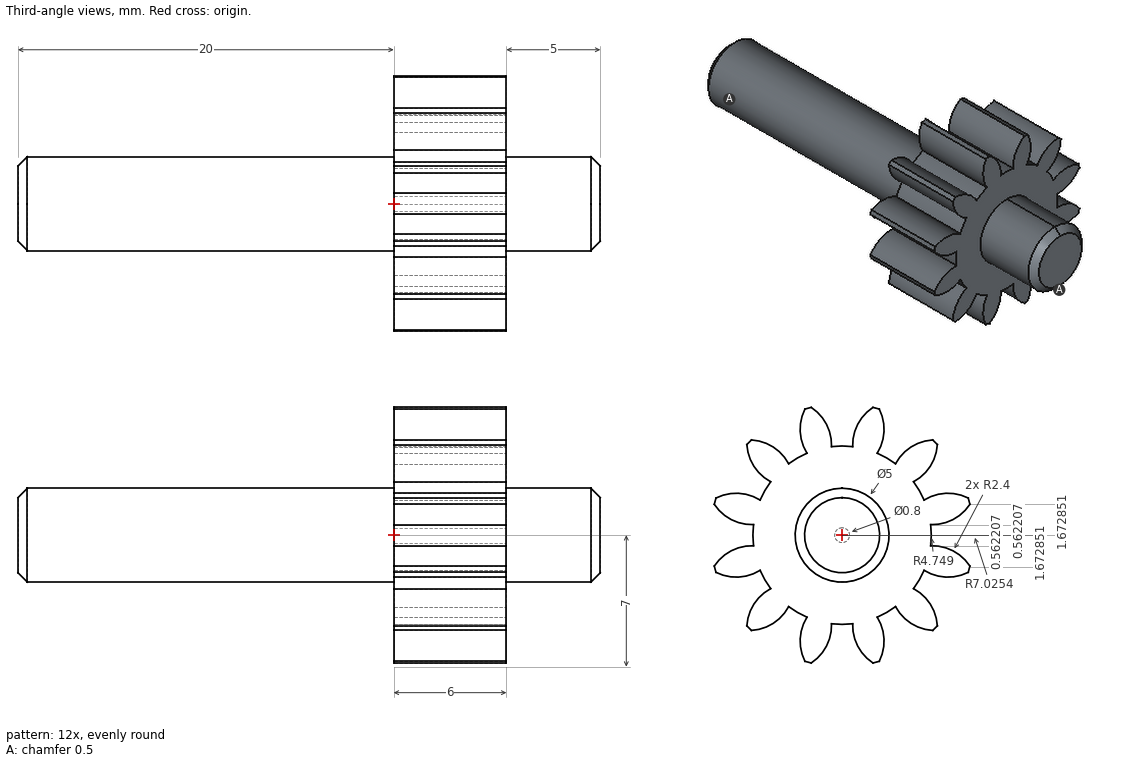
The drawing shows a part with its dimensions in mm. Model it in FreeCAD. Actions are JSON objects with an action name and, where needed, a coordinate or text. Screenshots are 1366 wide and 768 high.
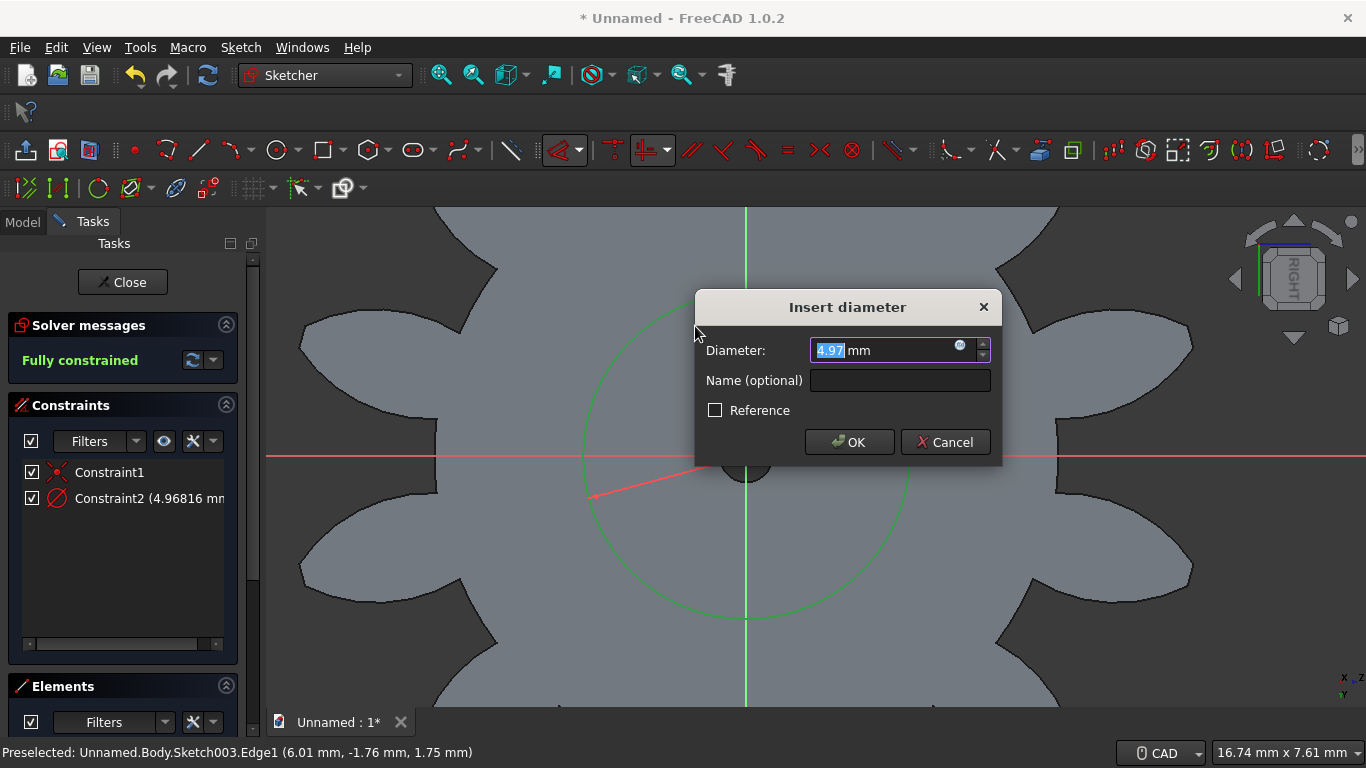
{"action": "type", "text": "5"}
{"action": "key", "text": "Return"}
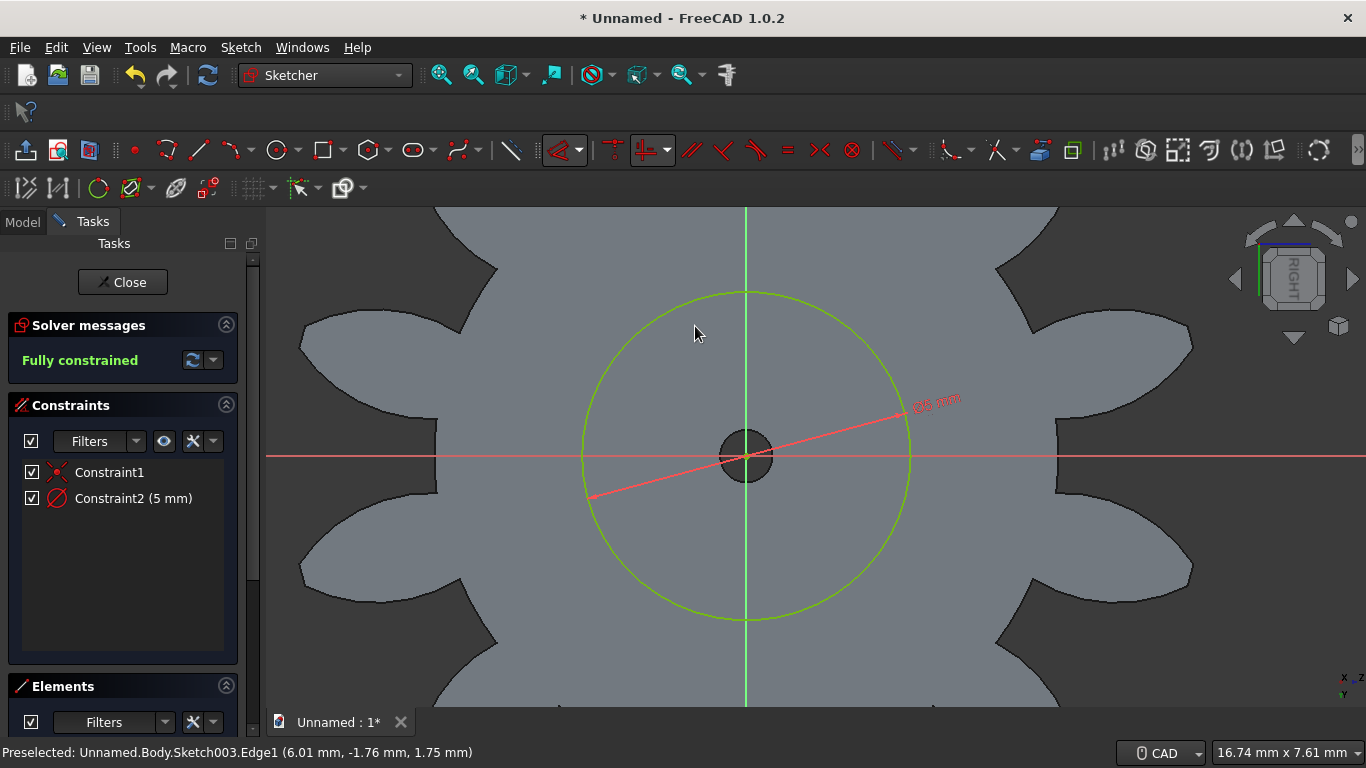
{"action": "left_click", "coordinate": [123, 282]}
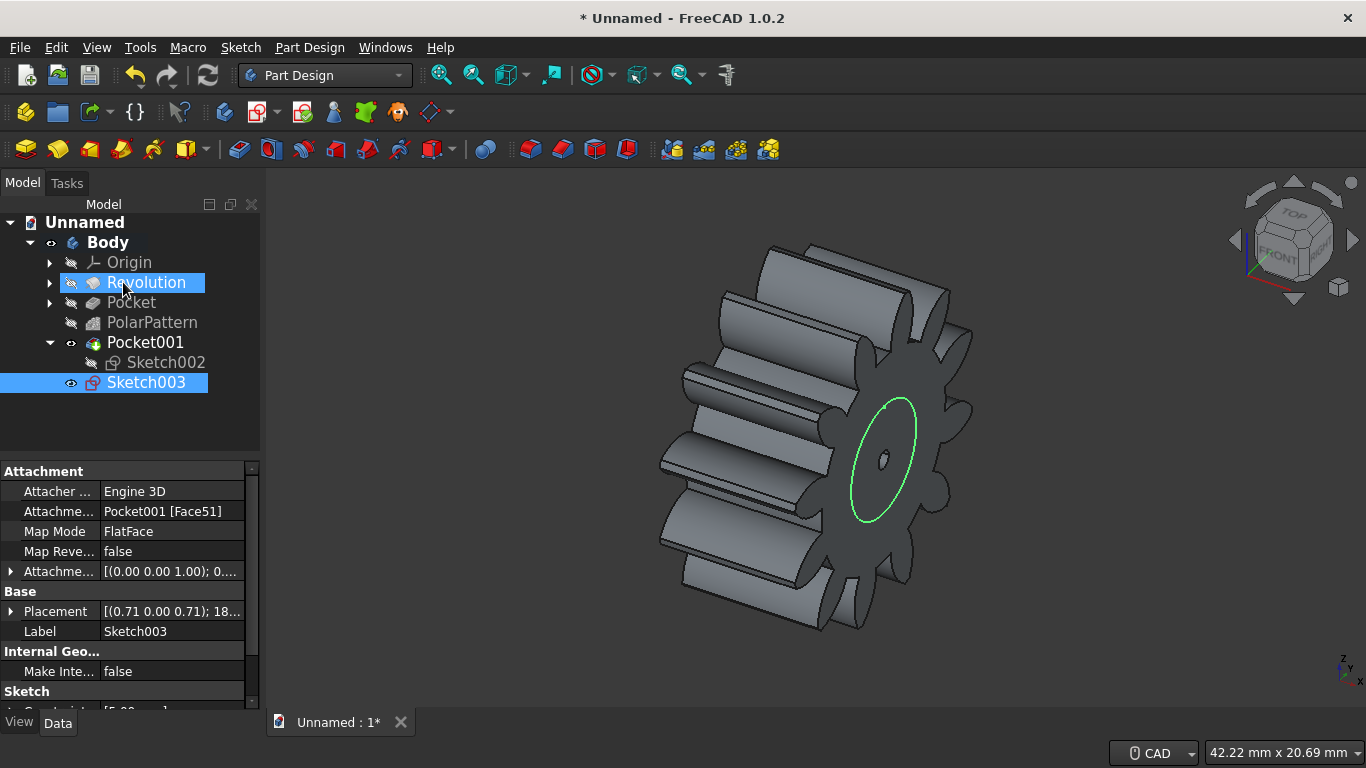
{"action": "left_click", "coordinate": [26, 150]}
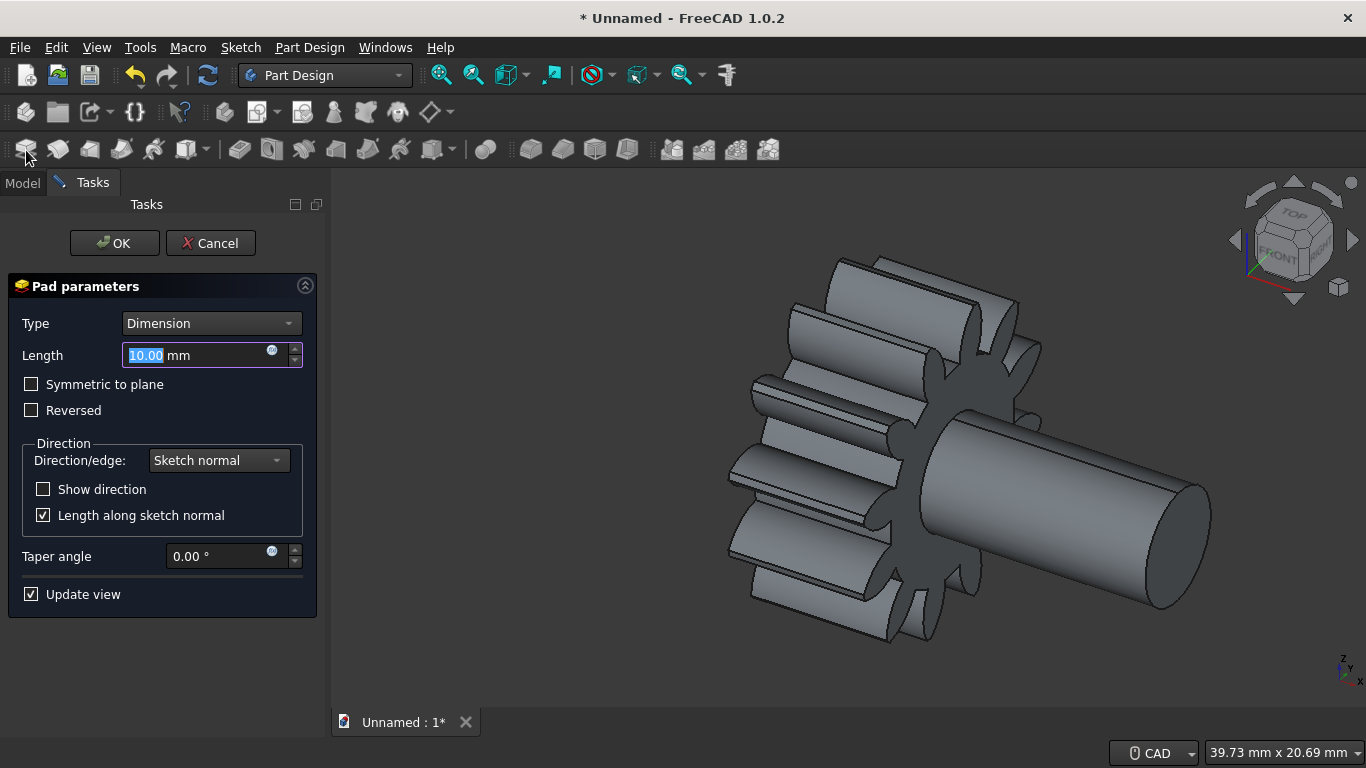
{"action": "type", "text": "5"}
{"action": "key", "text": "Tab"}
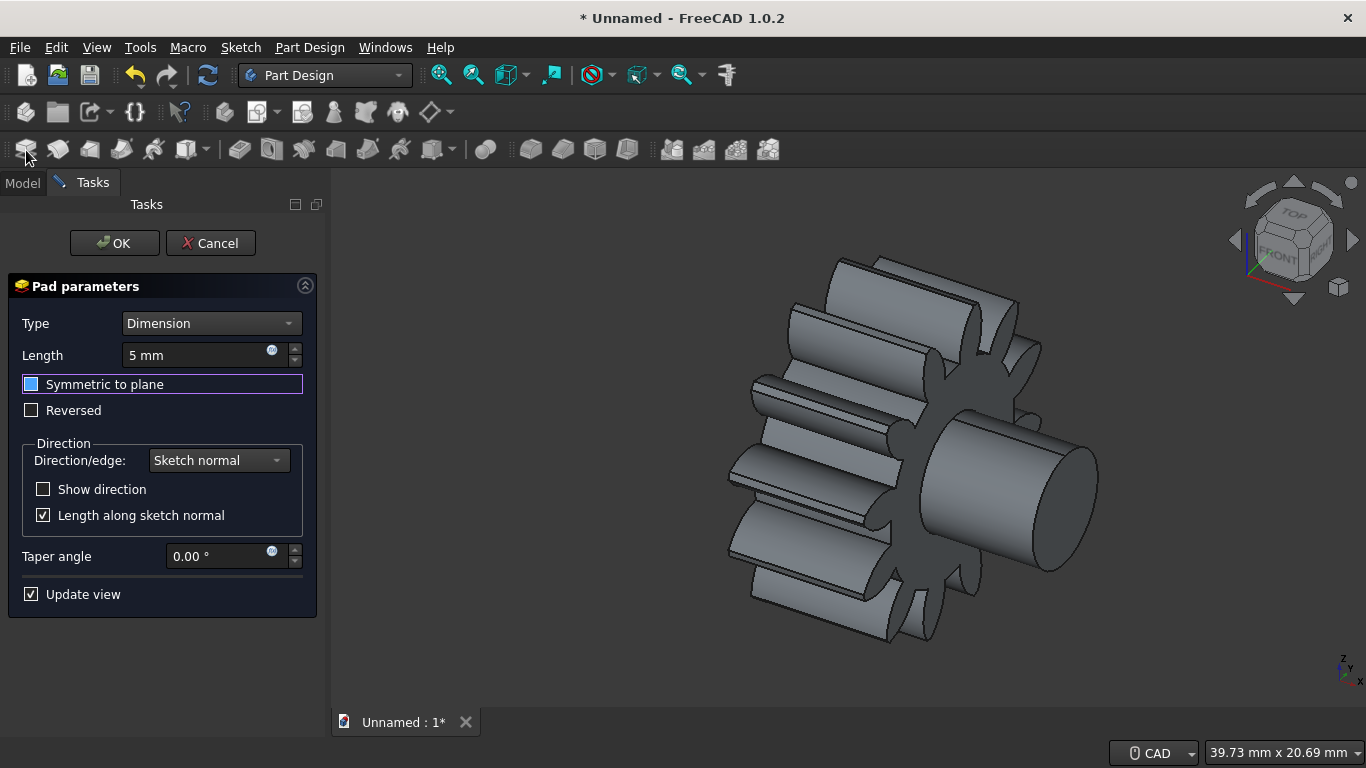
{"action": "left_click", "coordinate": [115, 243]}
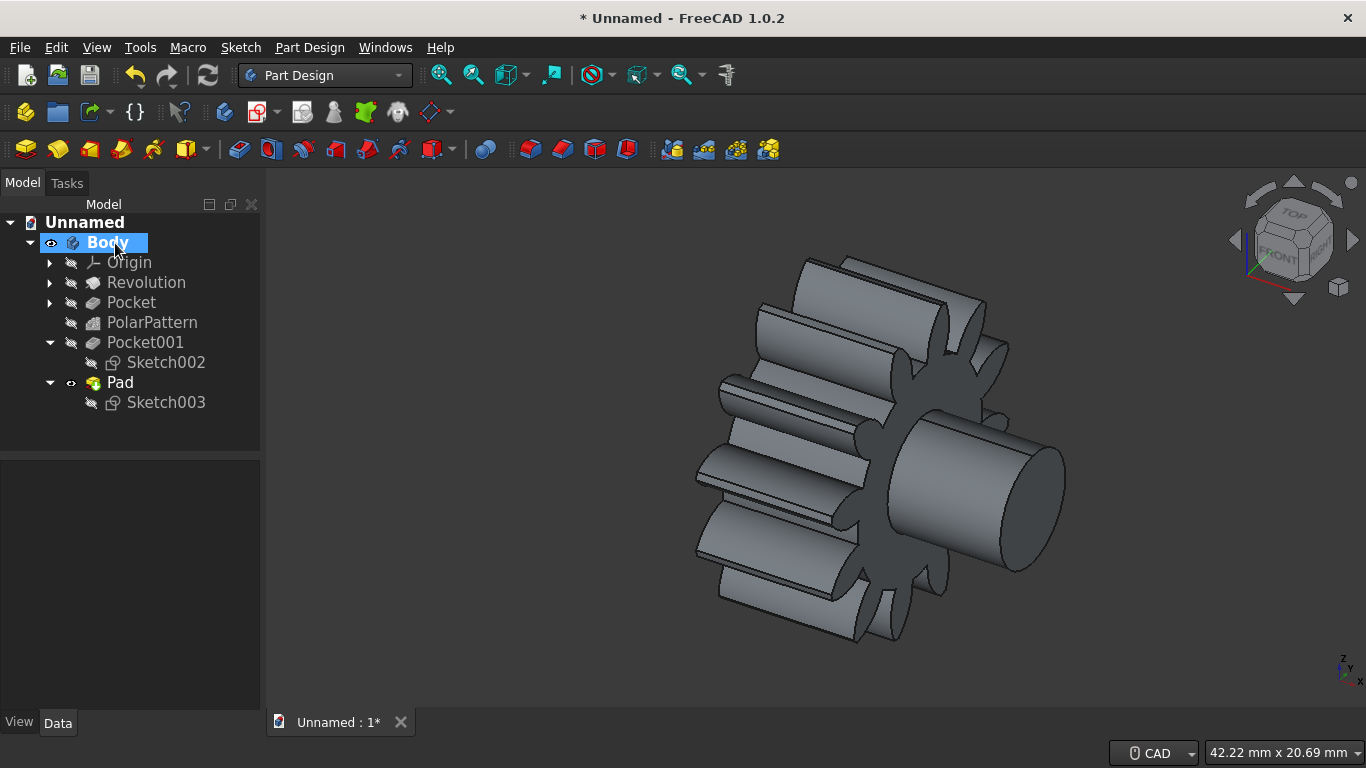
{"action": "left_click", "coordinate": [442, 76]}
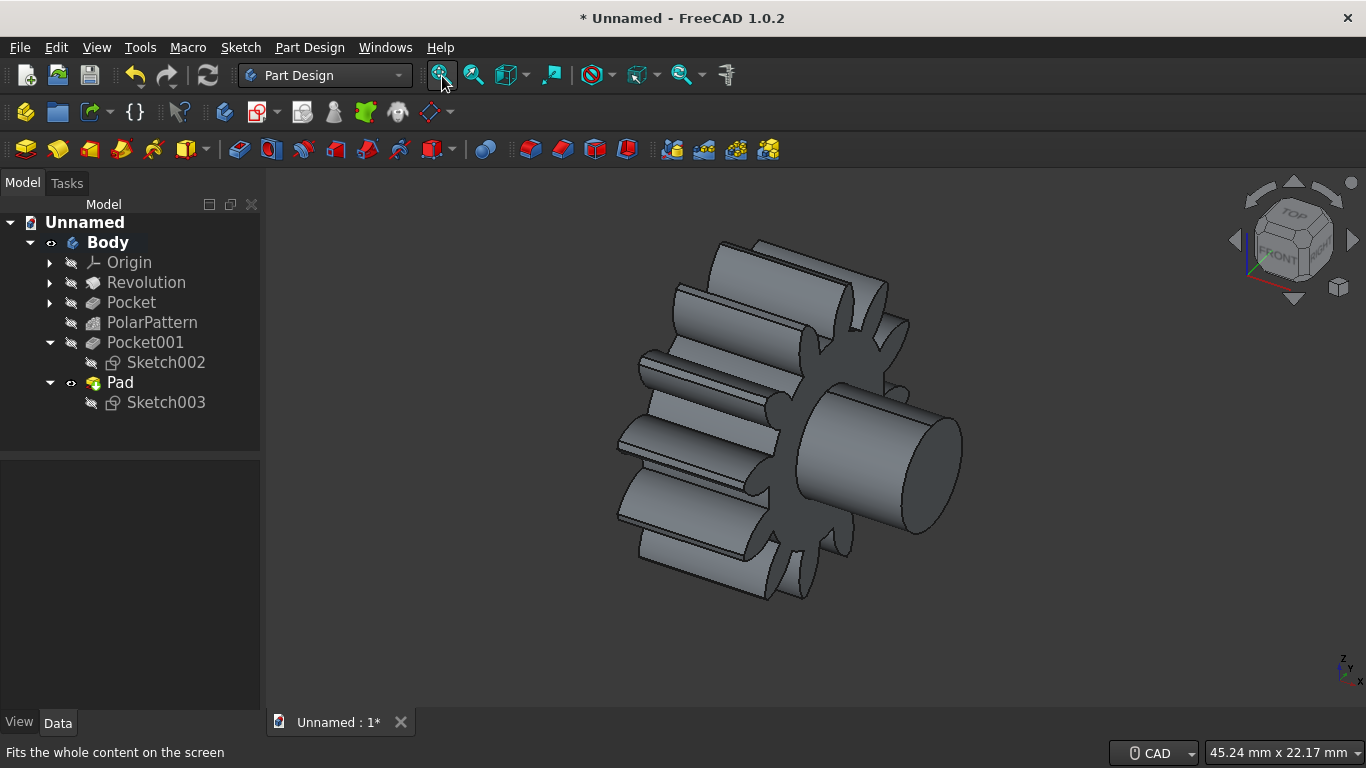
{"action": "left_click", "coordinate": [50, 263]}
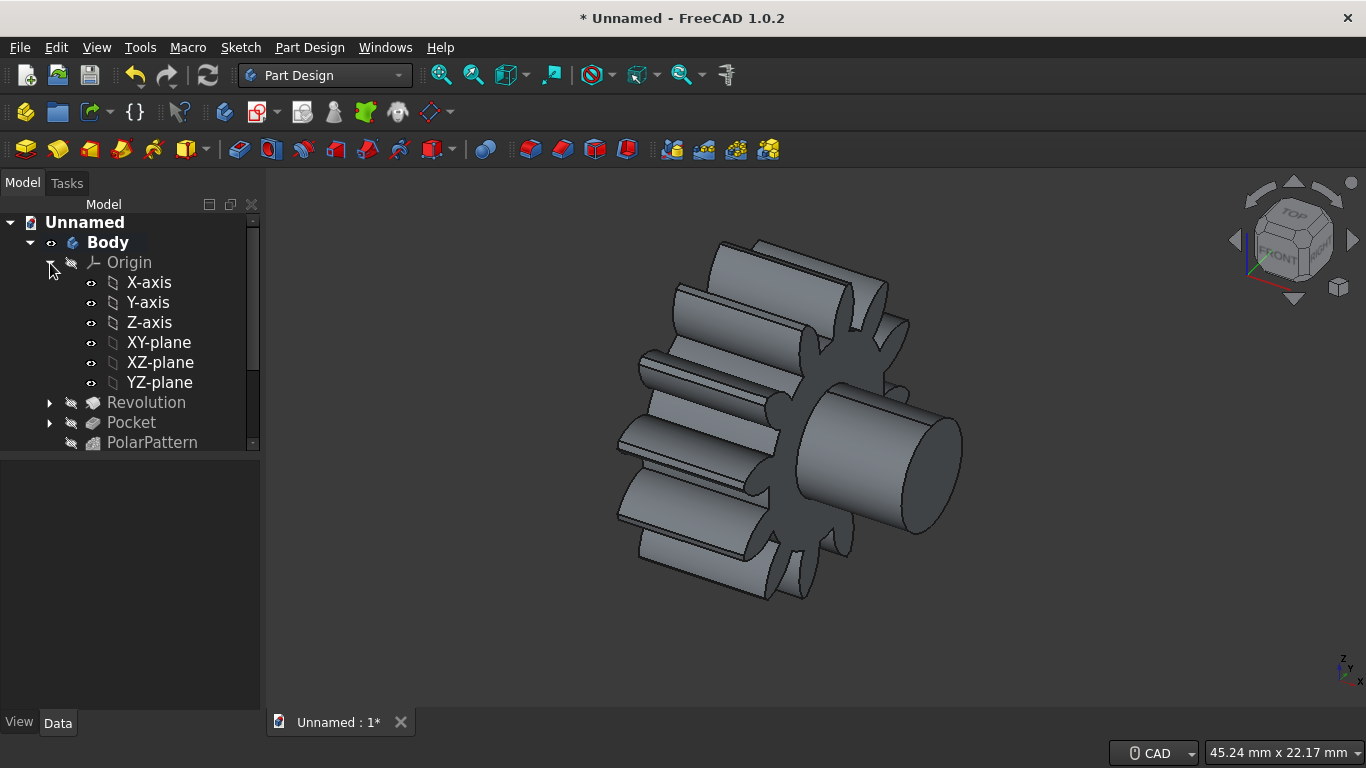
{"action": "left_click", "coordinate": [136, 383]}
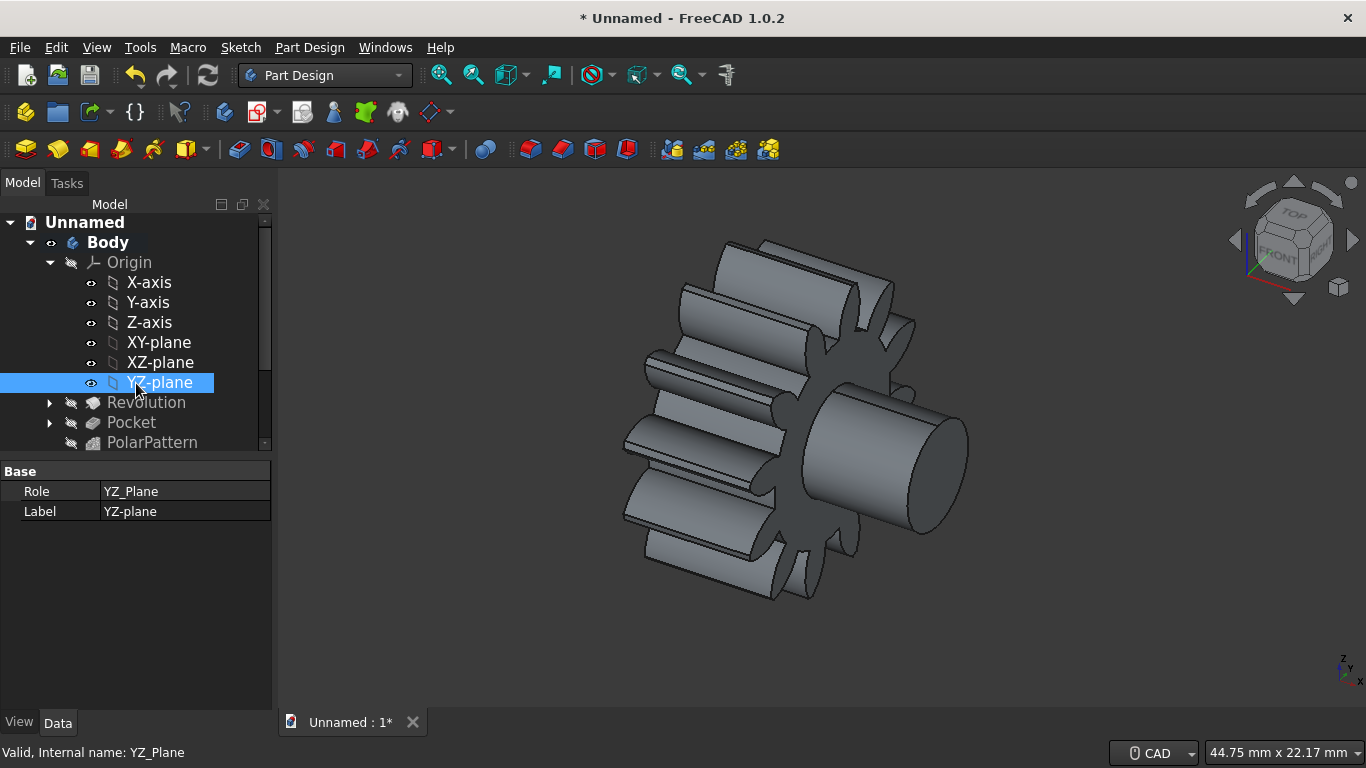
{"action": "left_click", "coordinate": [430, 112]}